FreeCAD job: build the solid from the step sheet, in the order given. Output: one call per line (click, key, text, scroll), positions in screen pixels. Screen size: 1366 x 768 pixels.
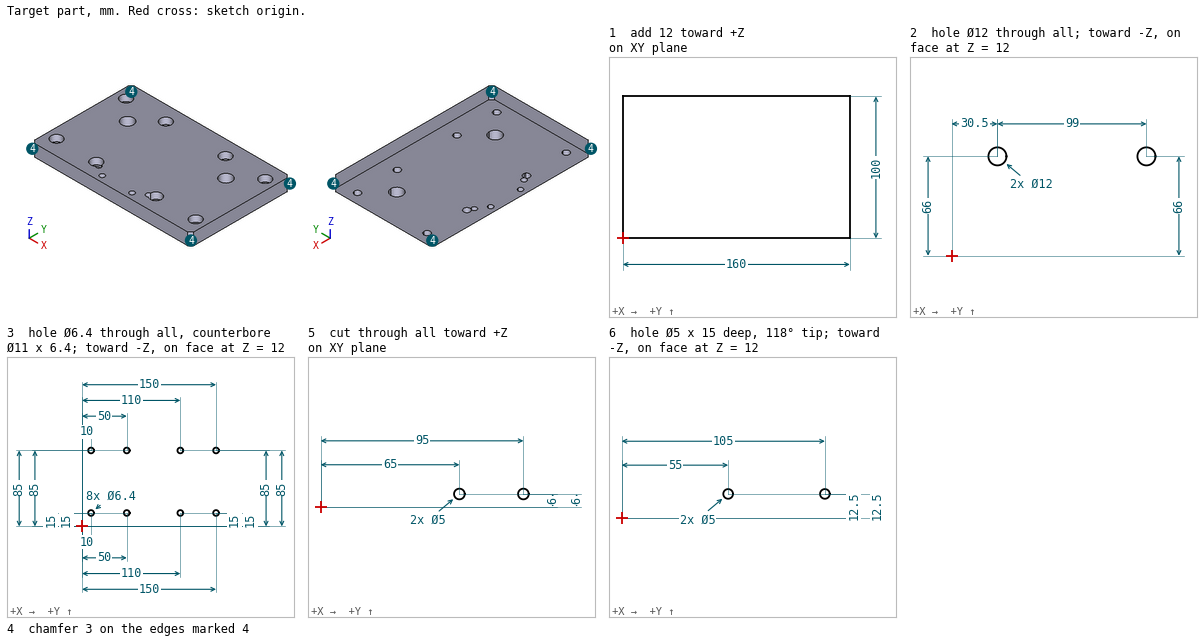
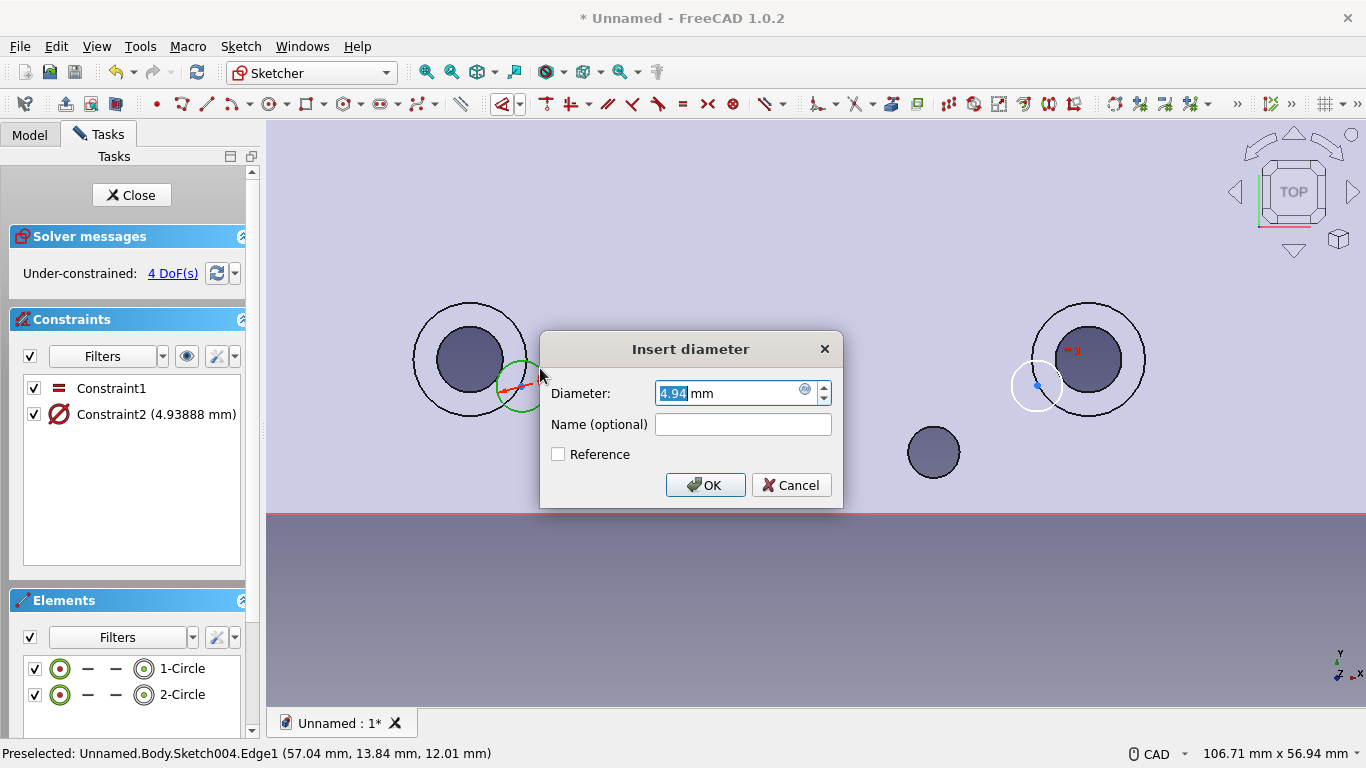
text(5)
key(Return)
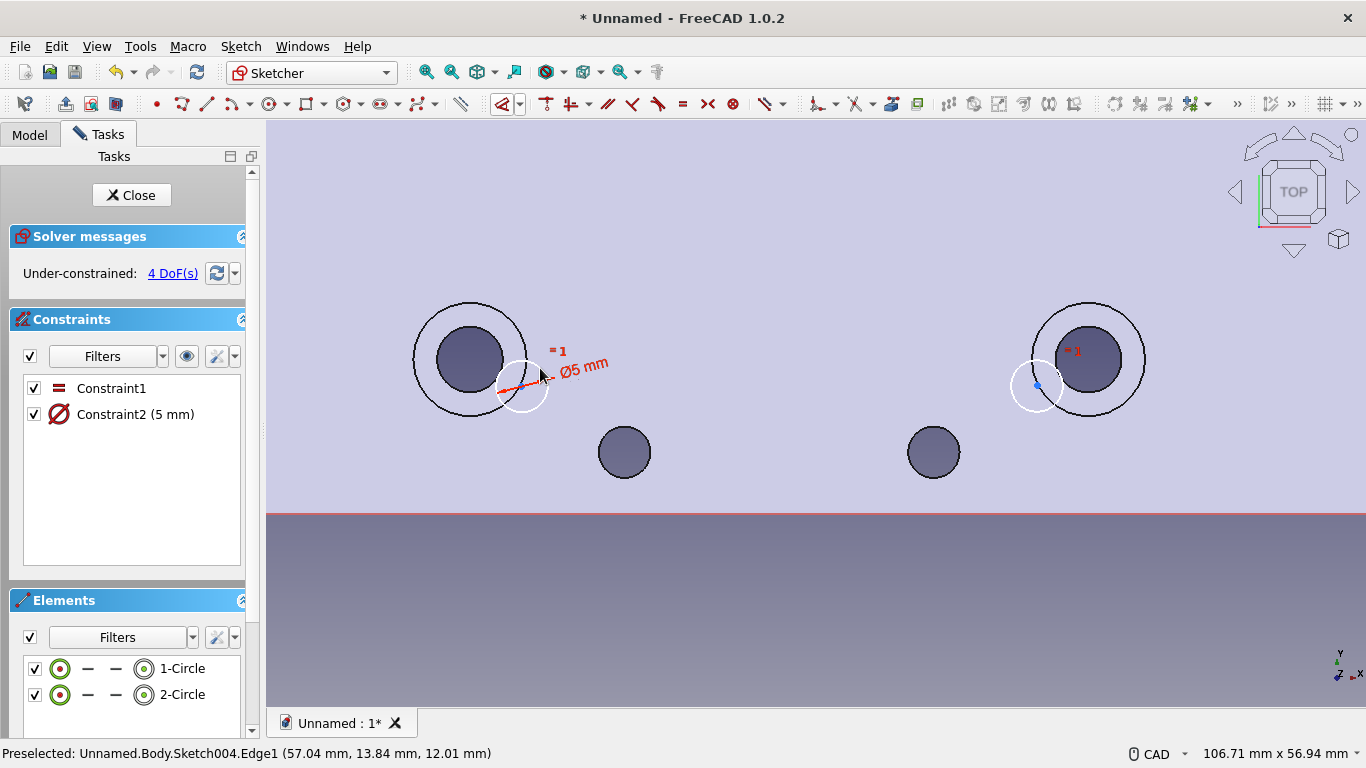
click(522, 386)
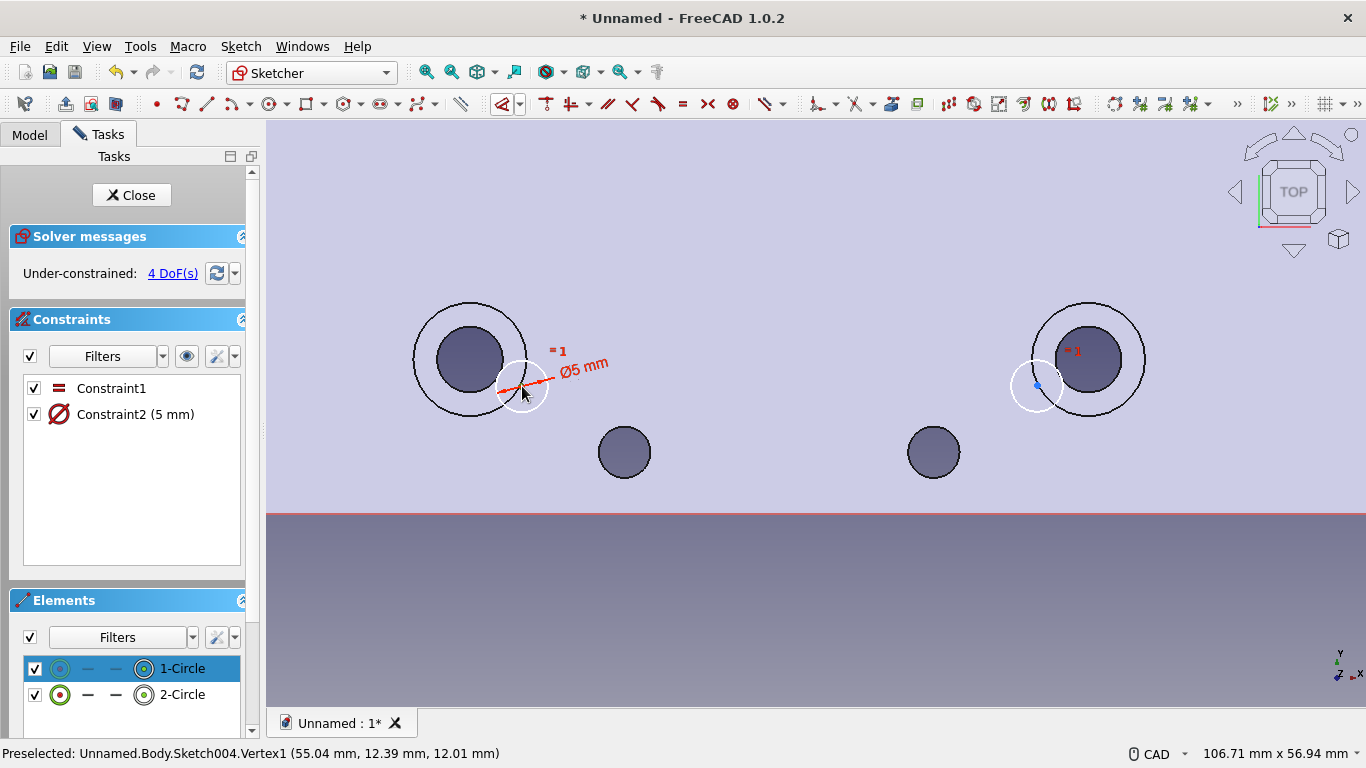
key(l)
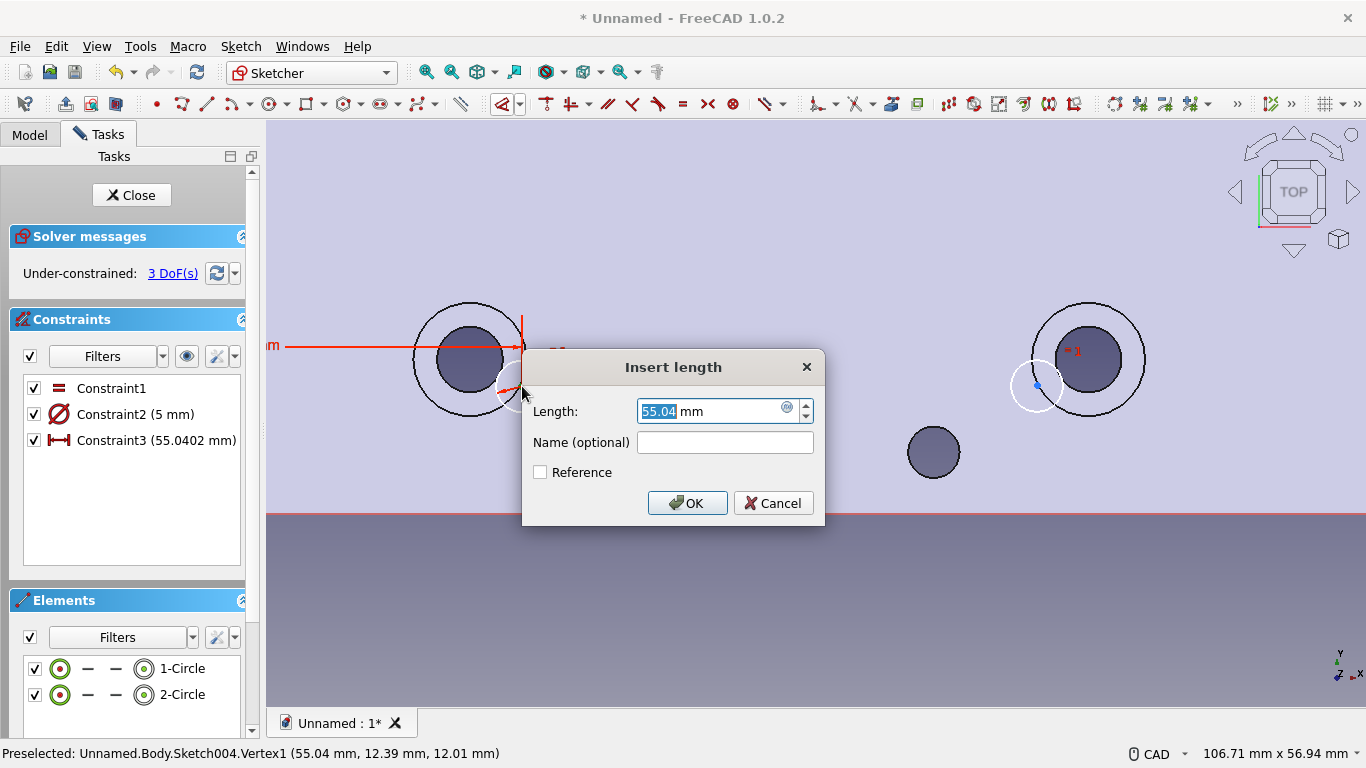
text(55)
key(Return)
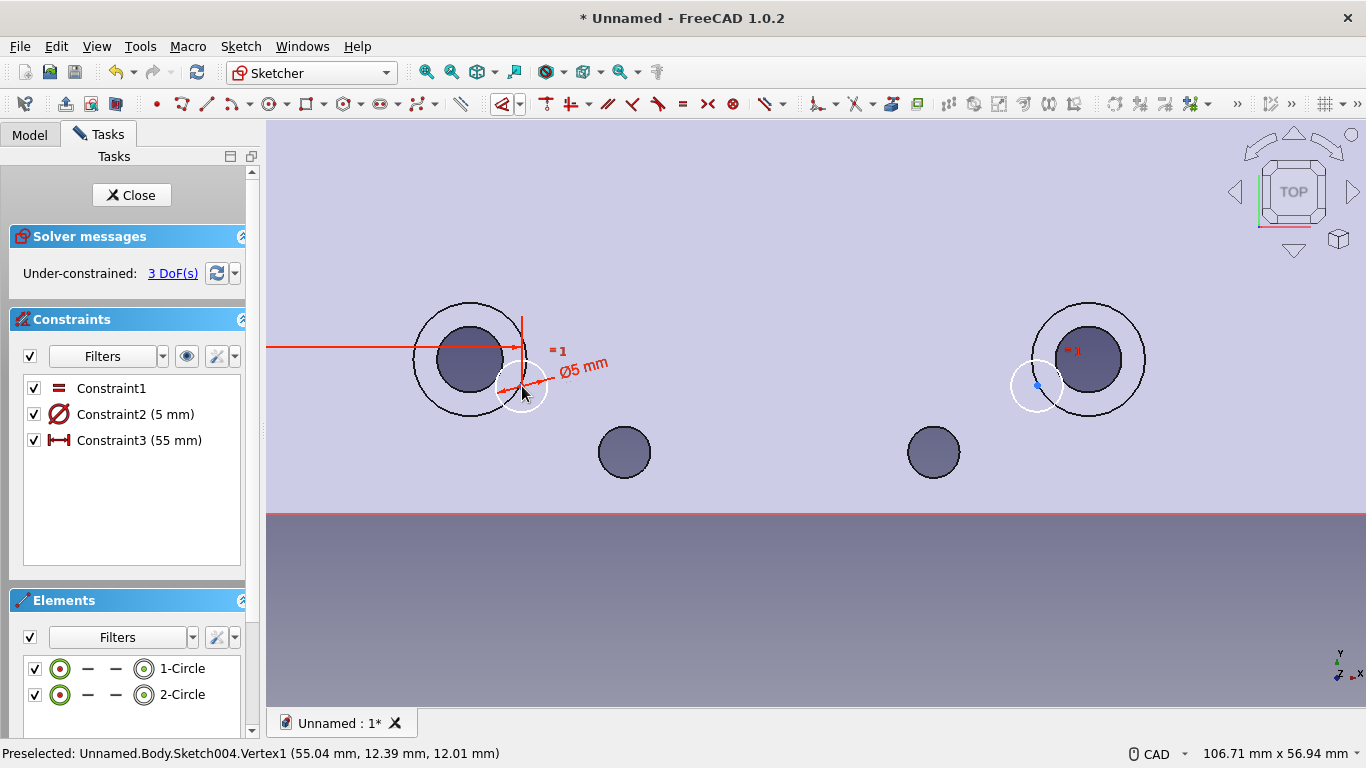
click(1037, 386)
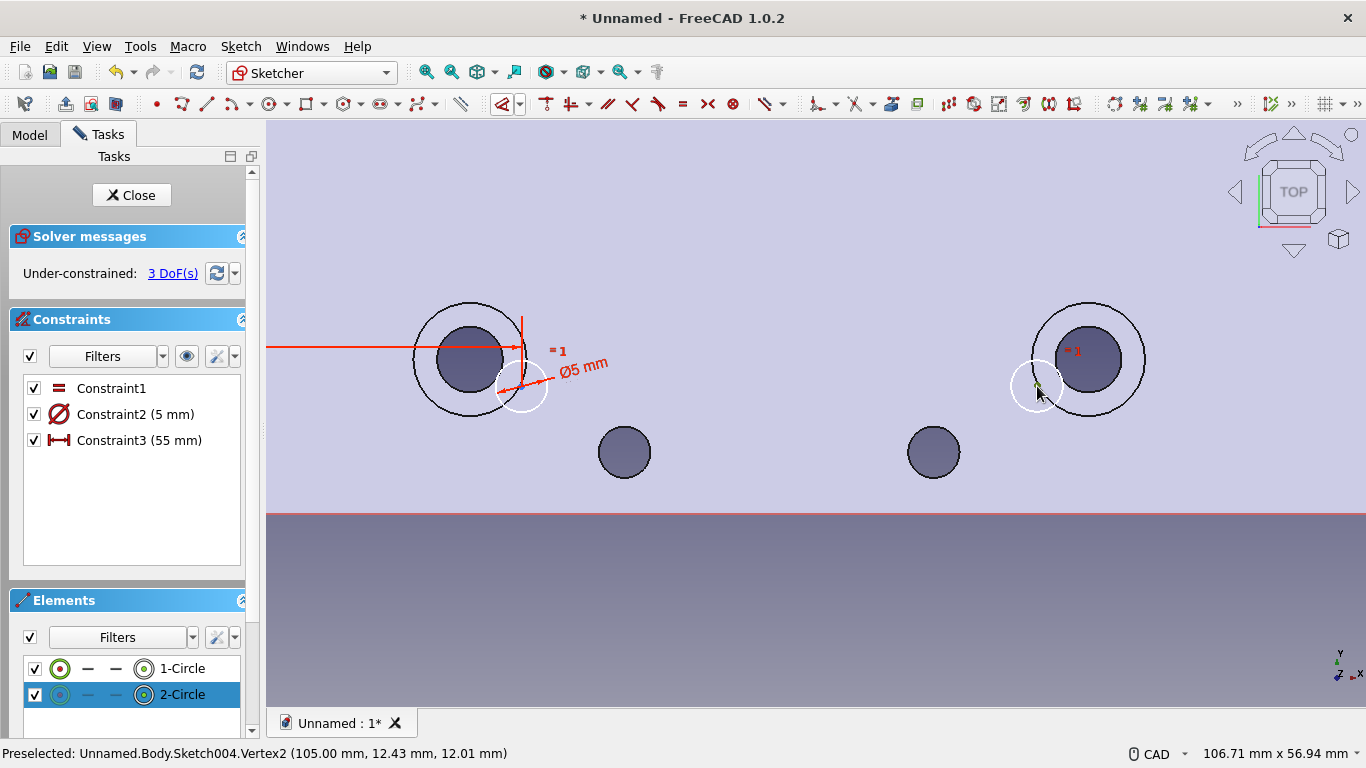
key(l)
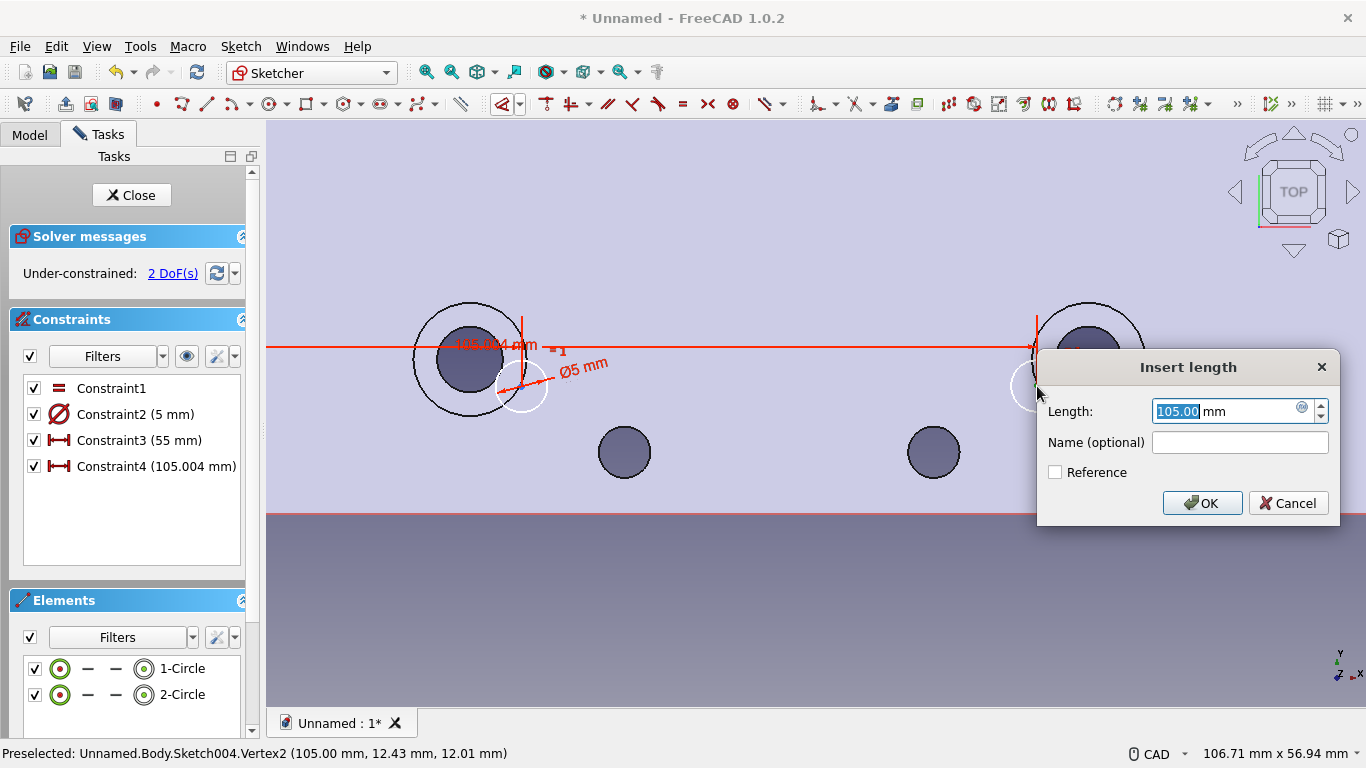
text(105)
key(Return)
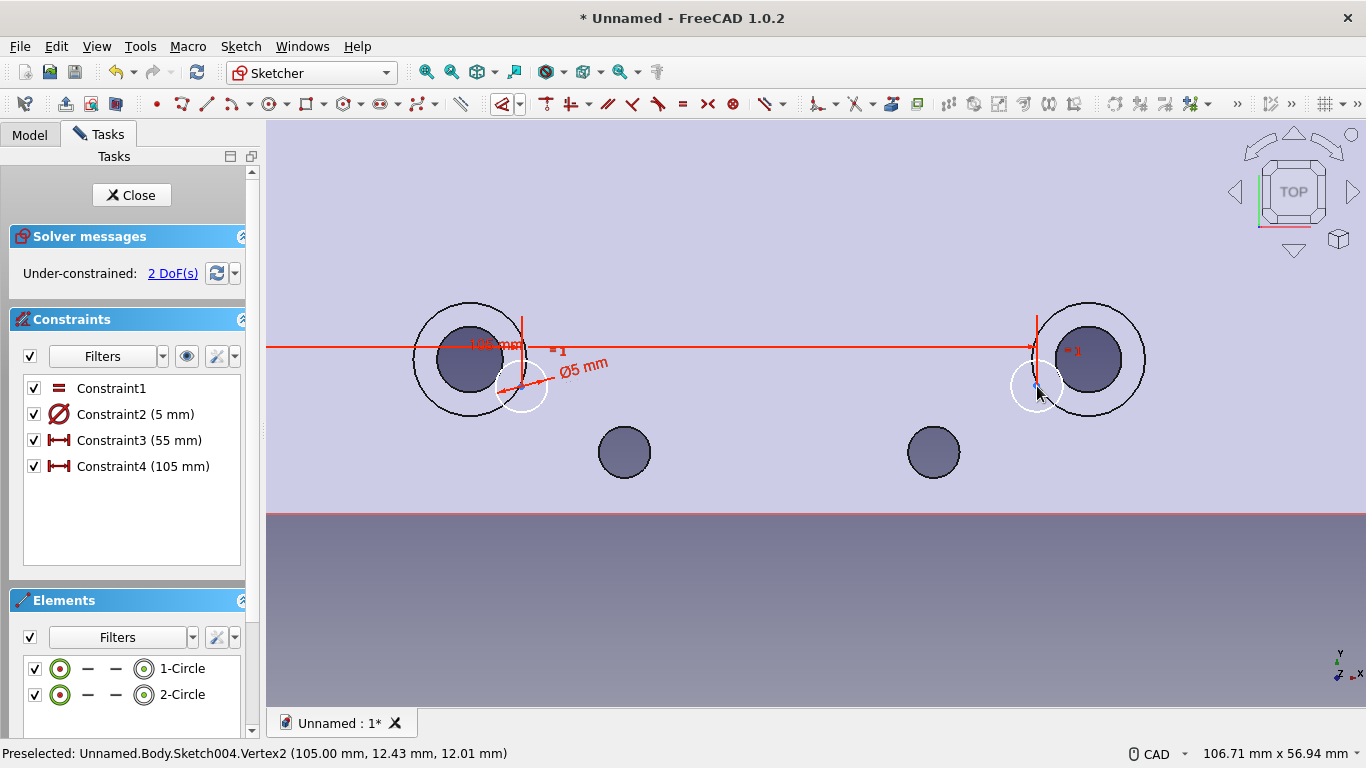
click(522, 386)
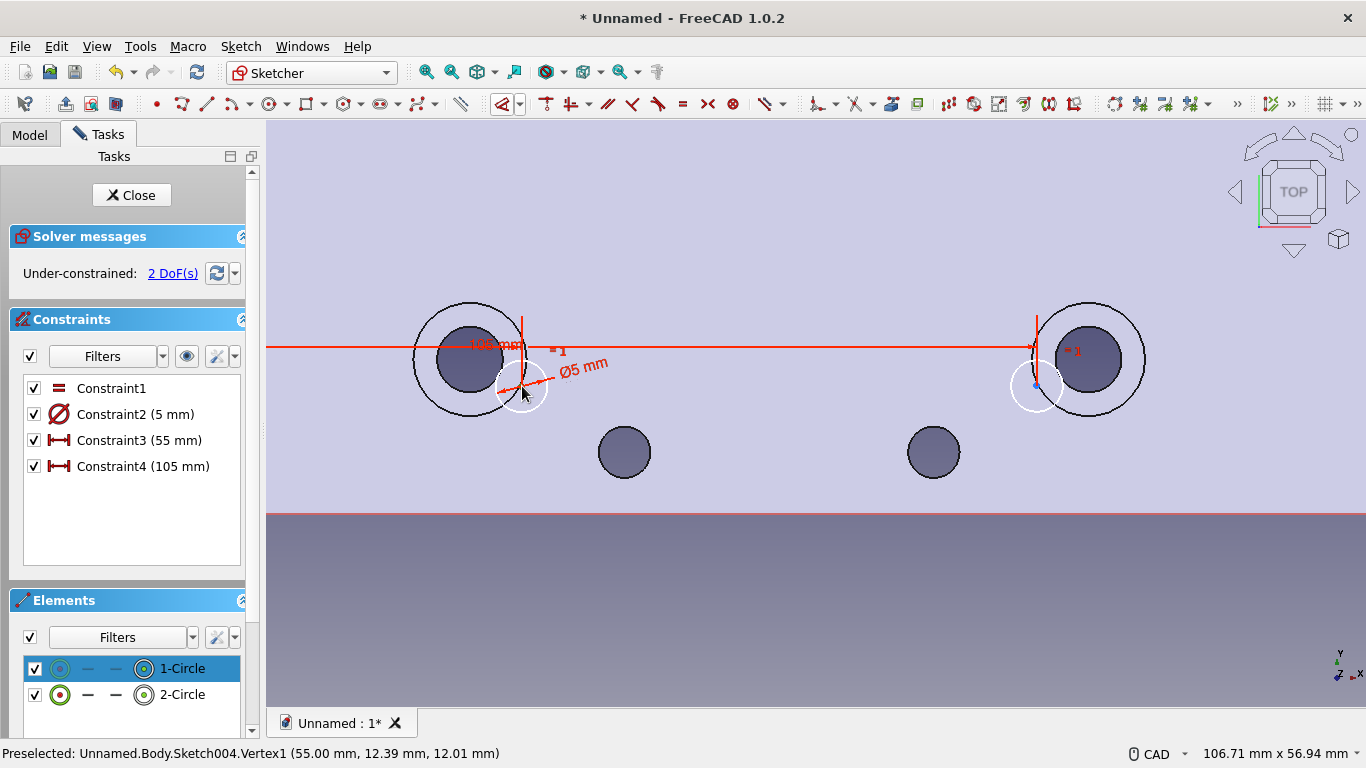
click(520, 104)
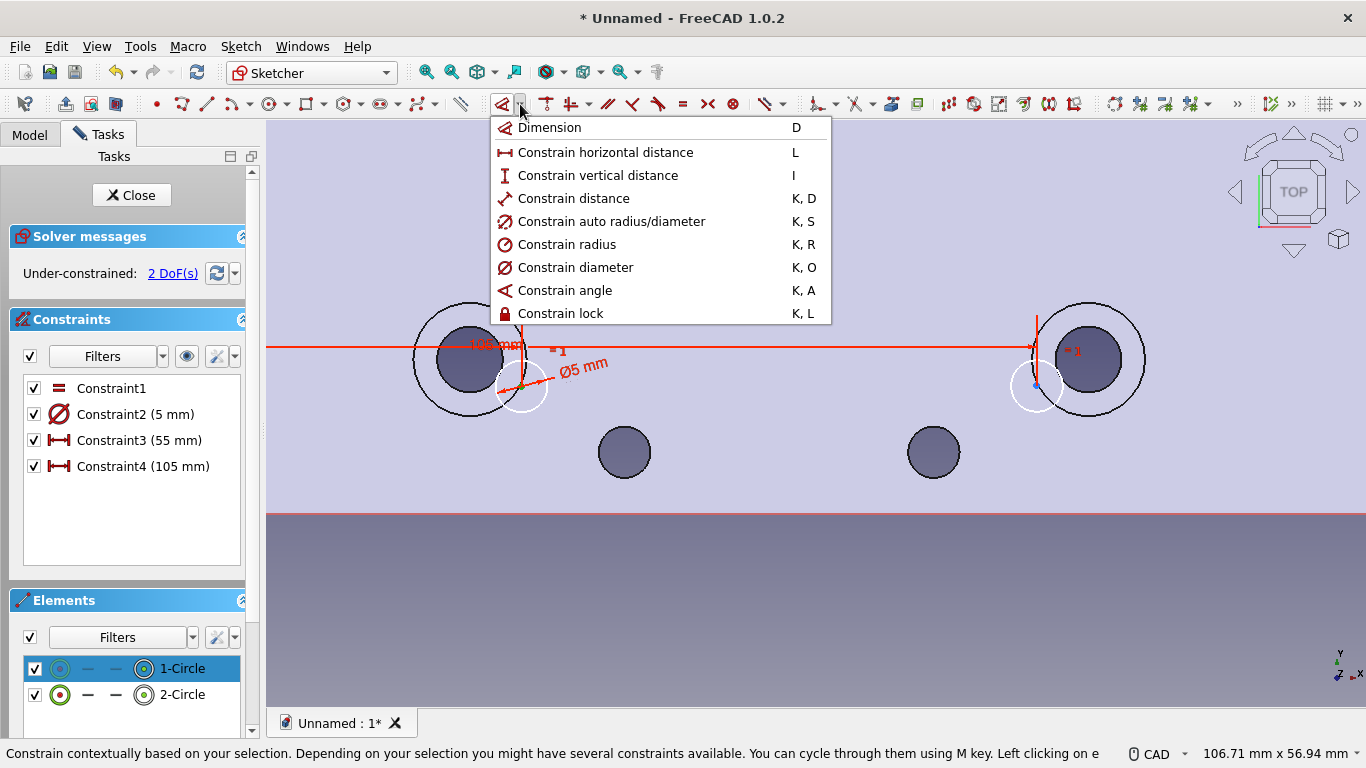
click(661, 176)